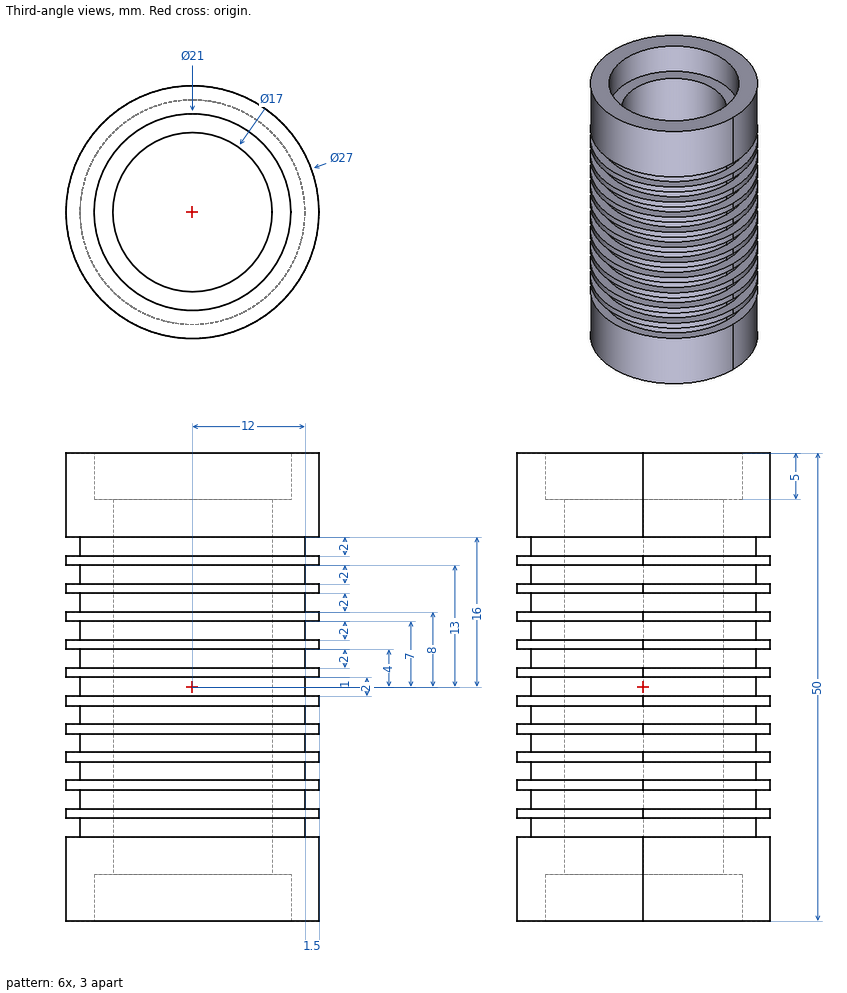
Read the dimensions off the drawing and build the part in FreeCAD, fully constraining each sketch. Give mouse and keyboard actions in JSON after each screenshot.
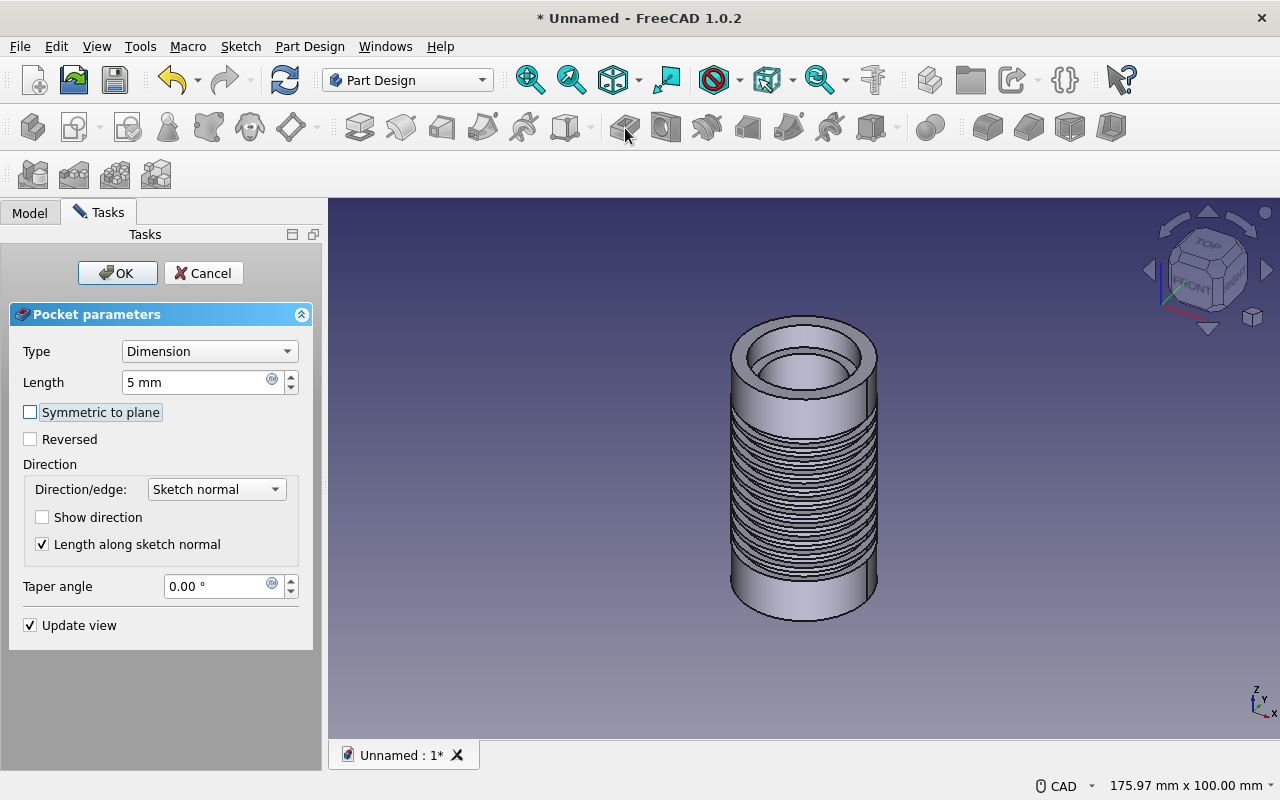
{"action": "left_click", "coordinate": [118, 273]}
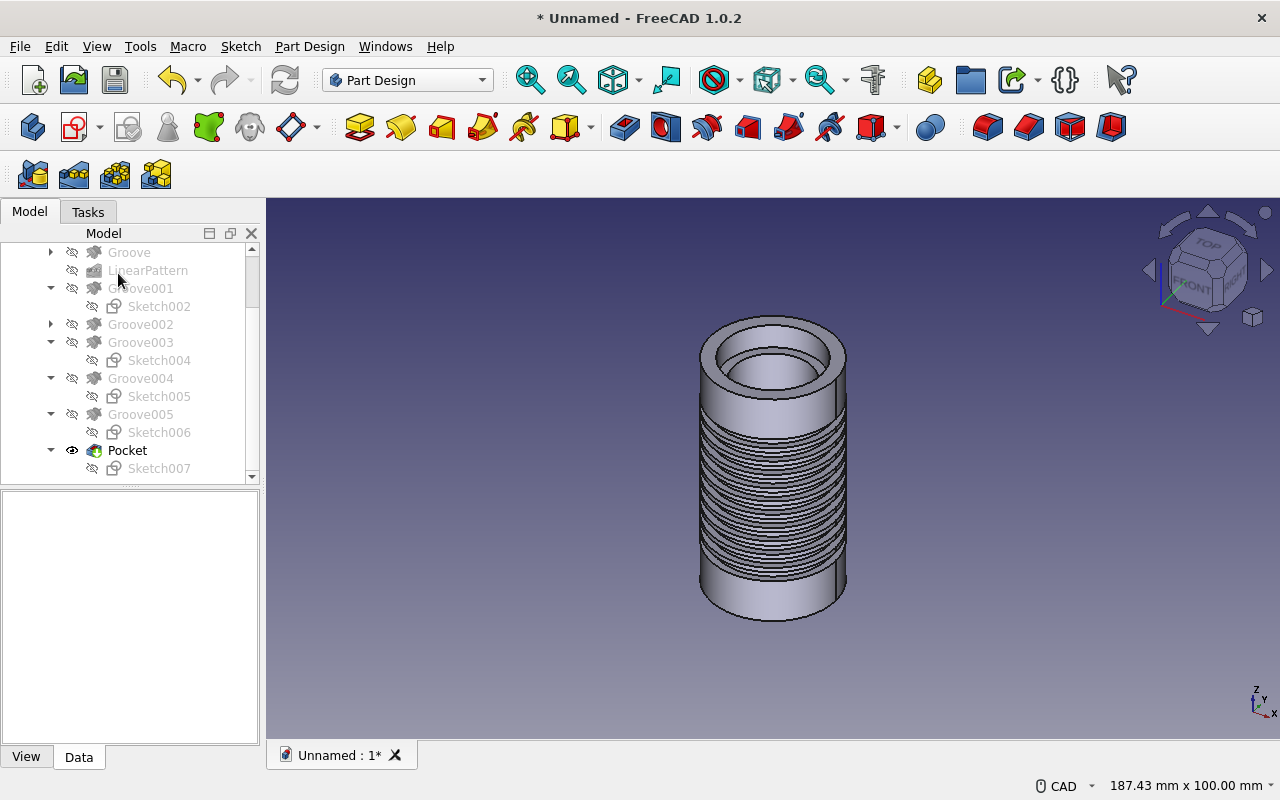
{"action": "left_click", "coordinate": [117, 450]}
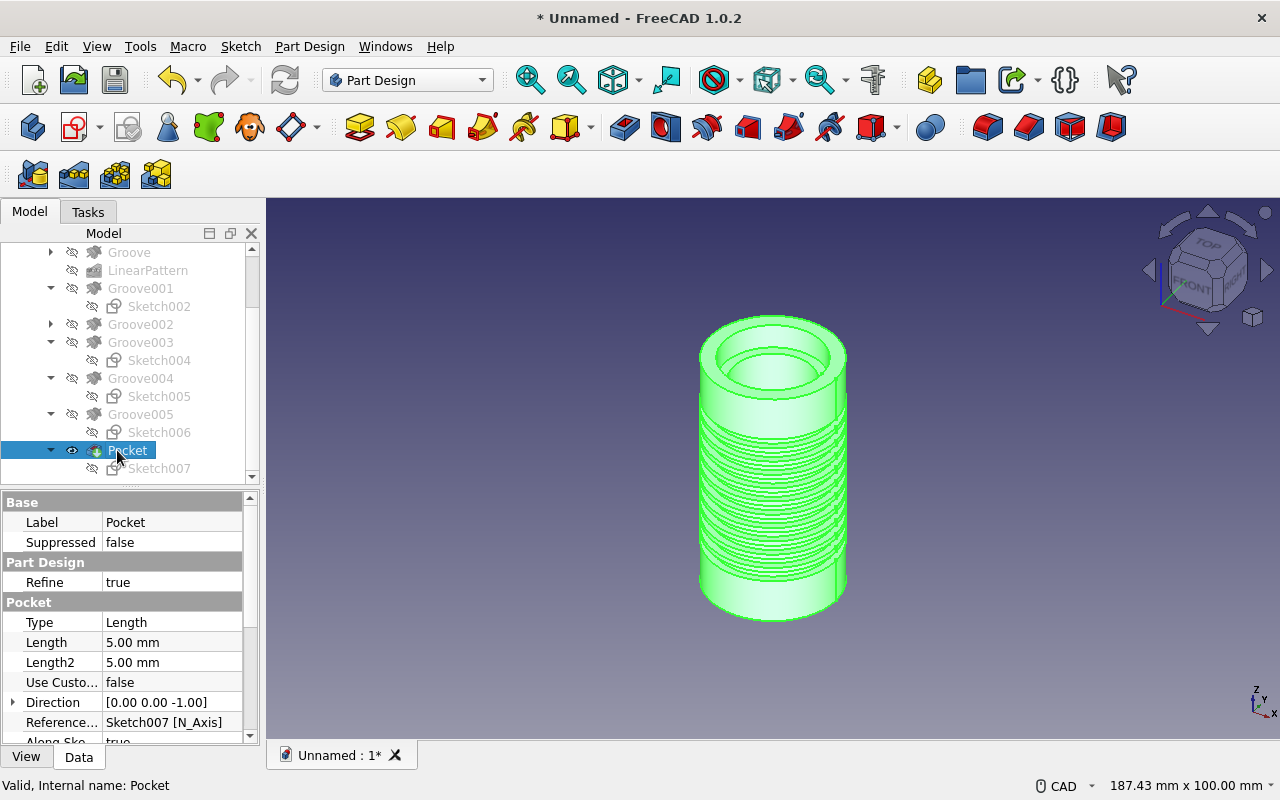
{"action": "left_click", "coordinate": [33, 174]}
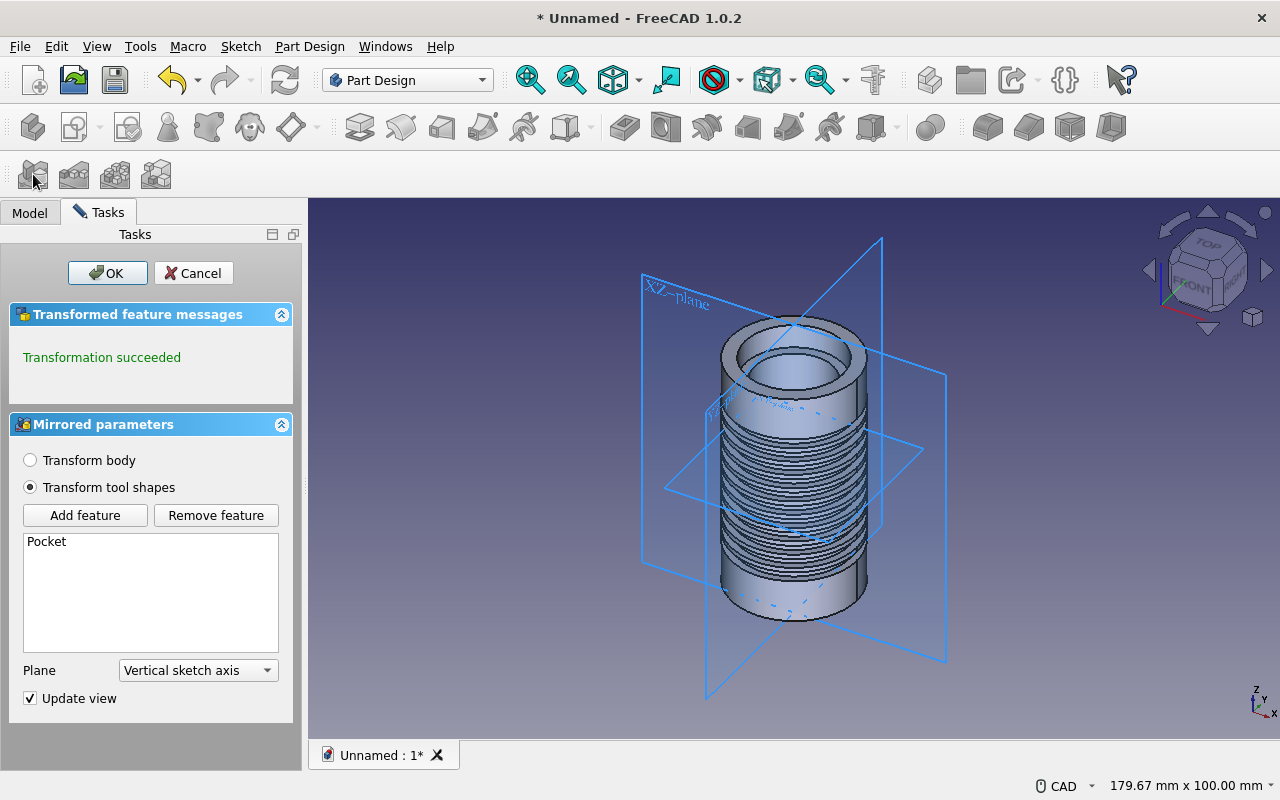
{"action": "left_click", "coordinate": [199, 670]}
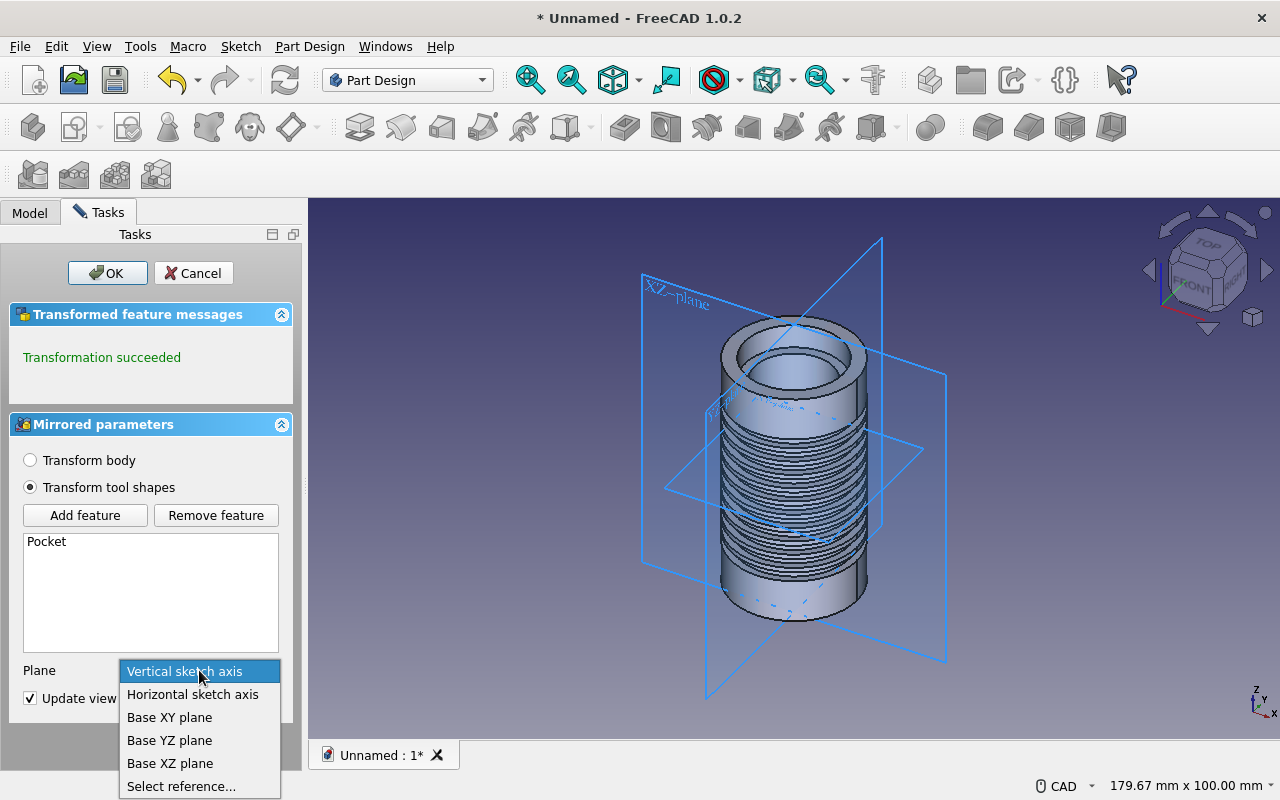
{"action": "left_click", "coordinate": [198, 718]}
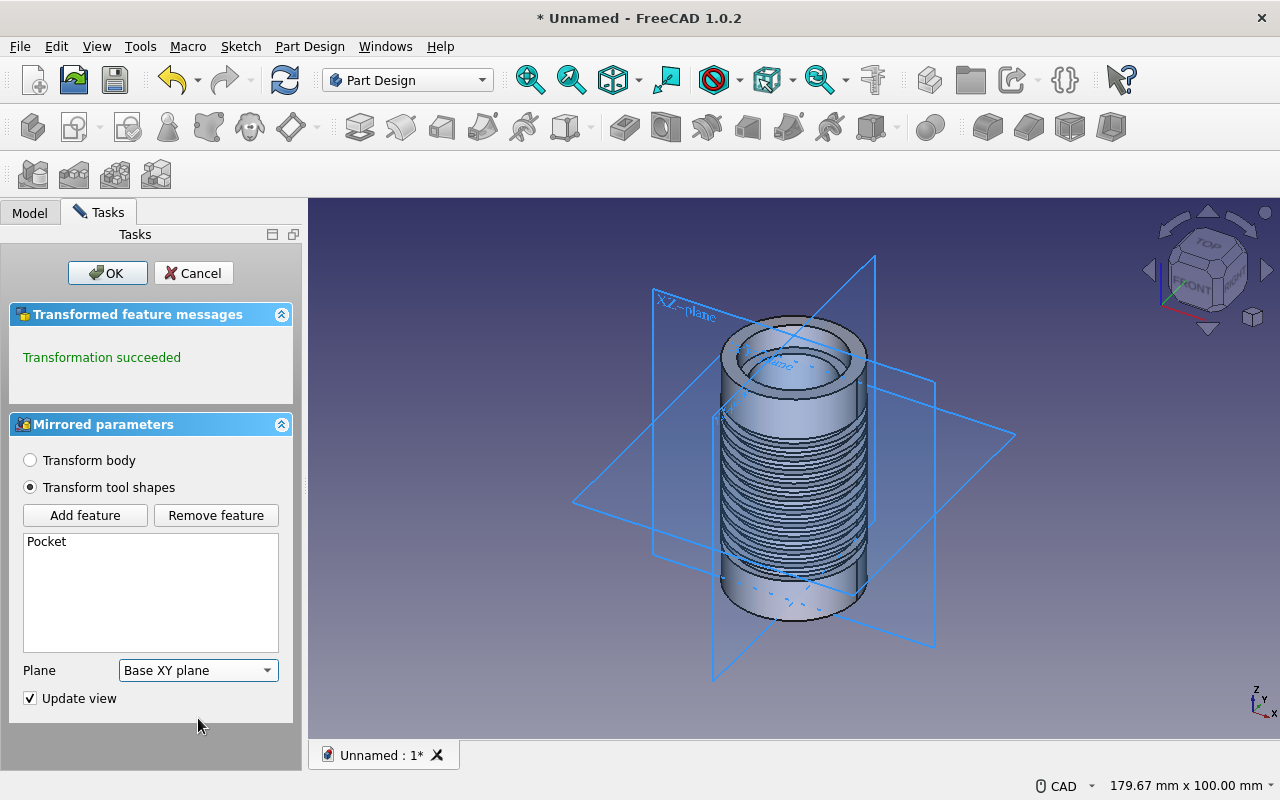
{"action": "left_click", "coordinate": [108, 273]}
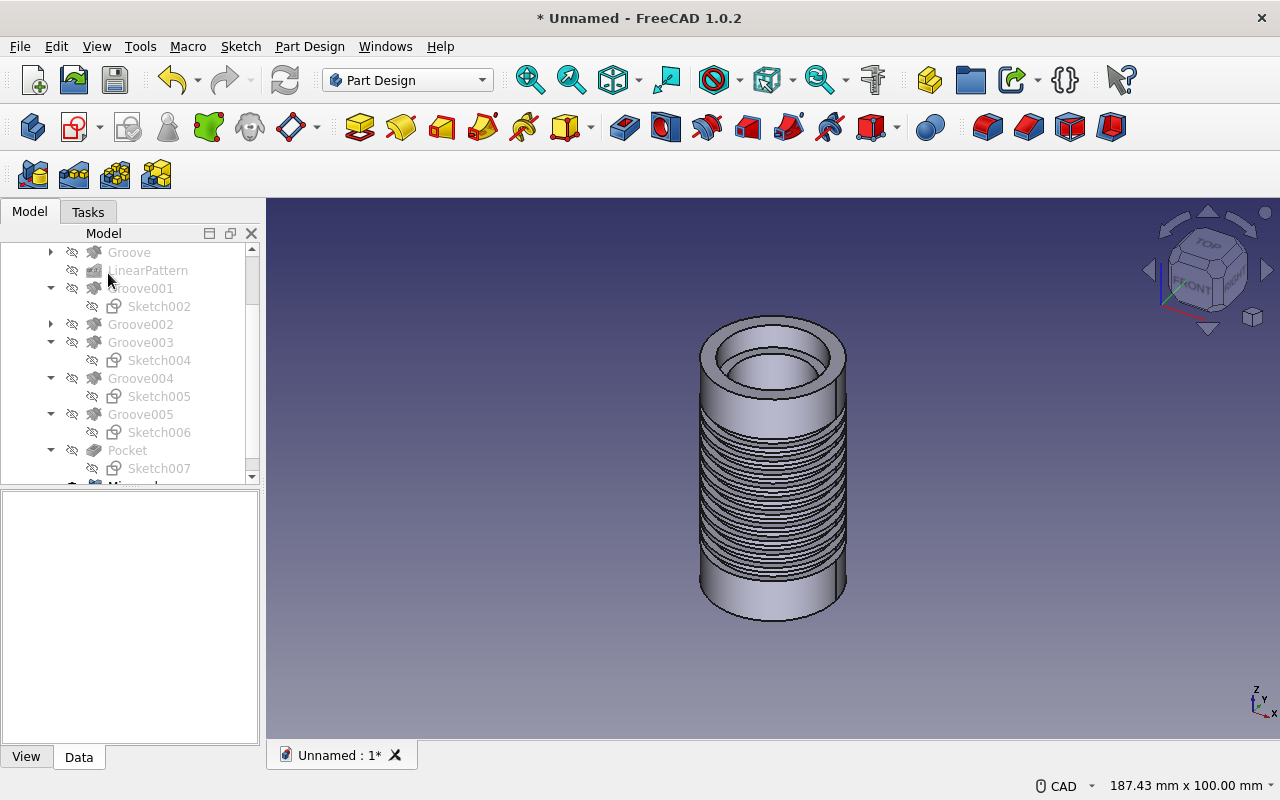
{"action": "key", "text": "0"}